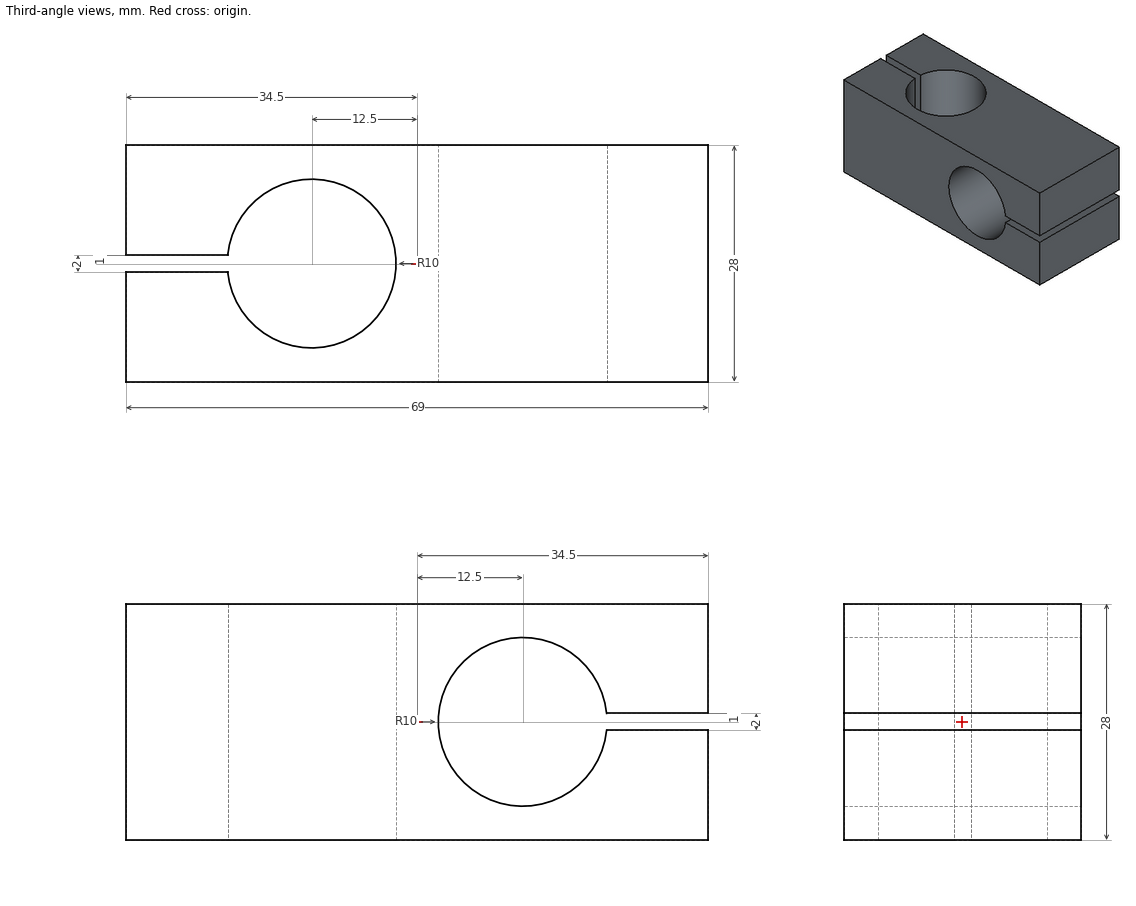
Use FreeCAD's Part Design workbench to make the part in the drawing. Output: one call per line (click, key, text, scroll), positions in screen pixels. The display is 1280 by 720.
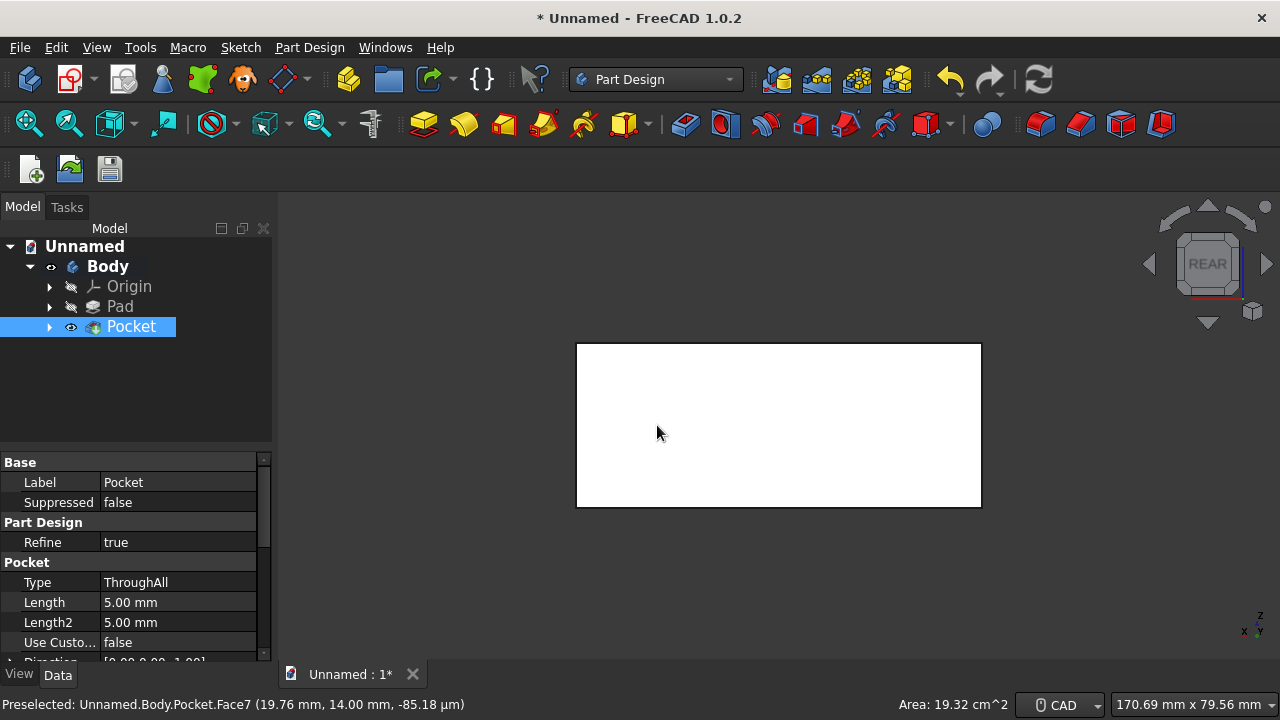
click(70, 80)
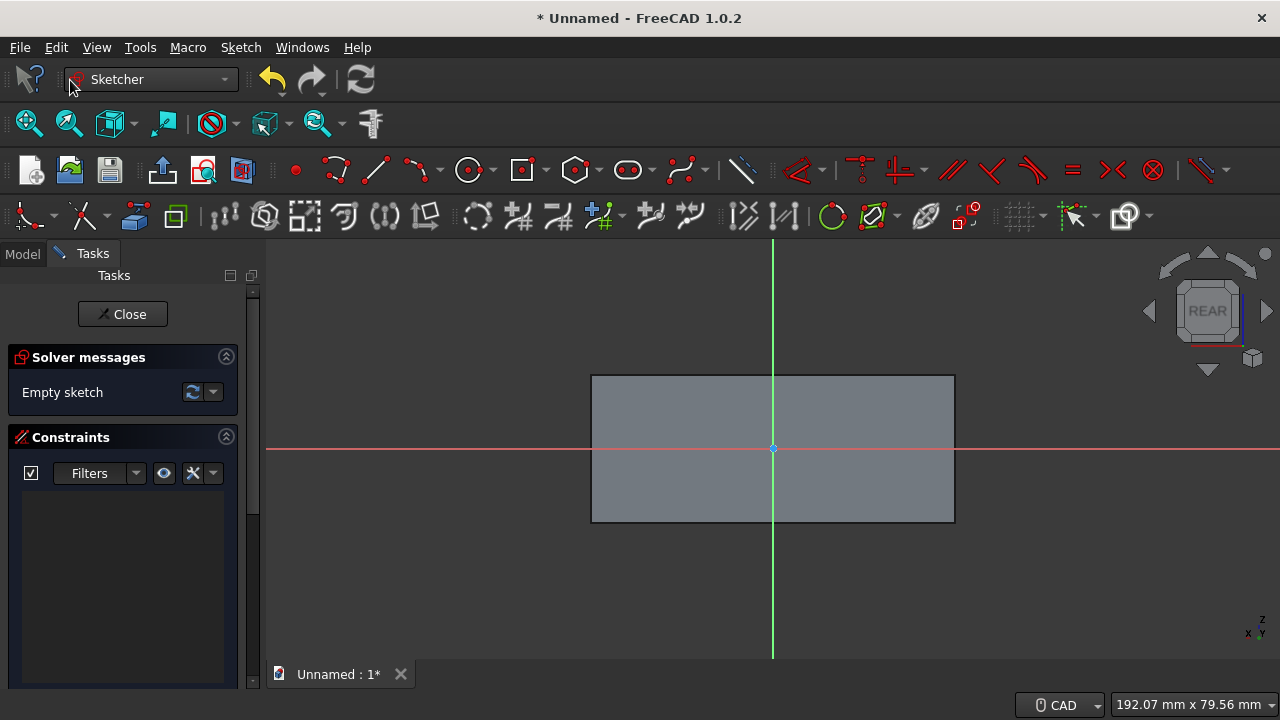
scroll(672, 449, up, 6)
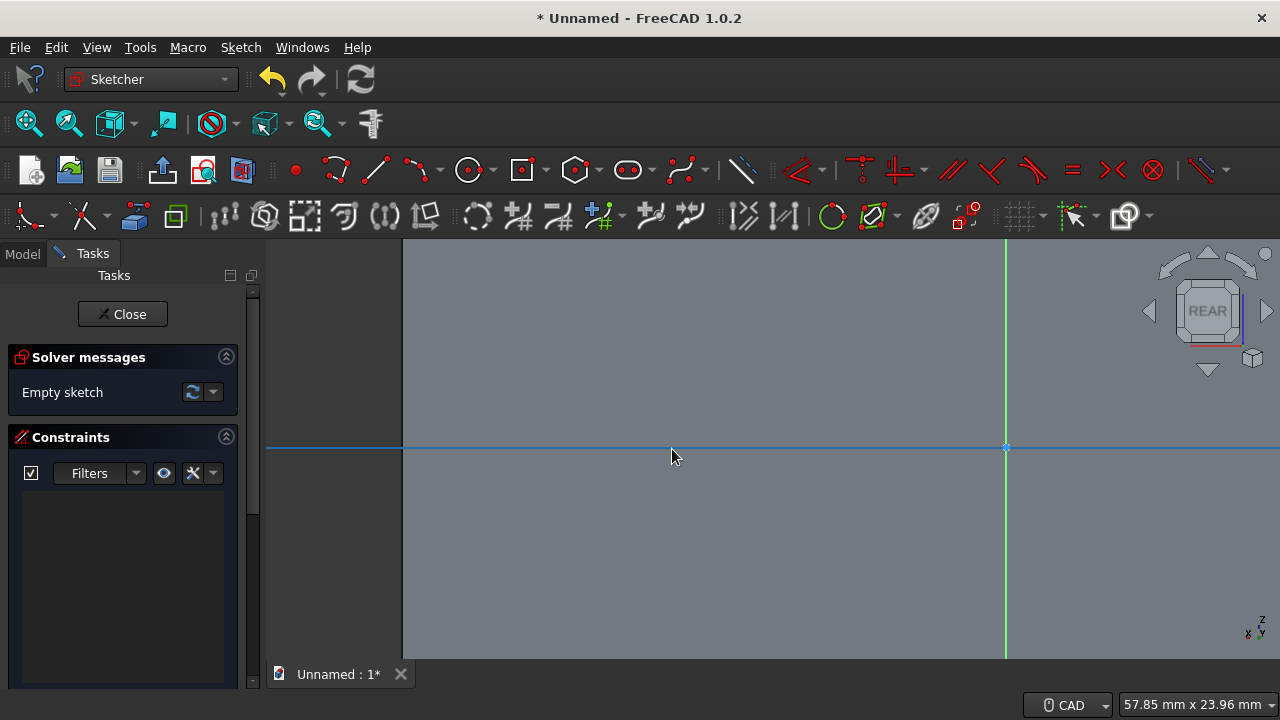
key(g)
key(m)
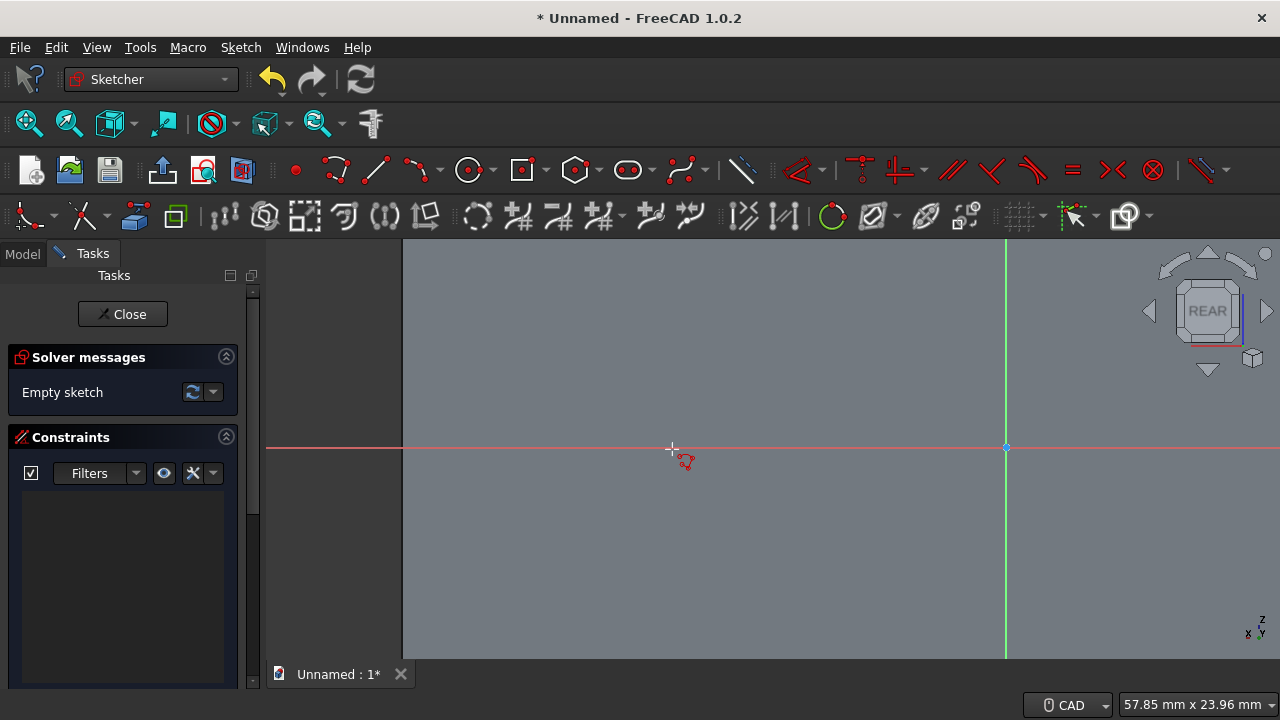
click(613, 430)
click(402, 430)
click(402, 465)
click(613, 465)
right_click(613, 465)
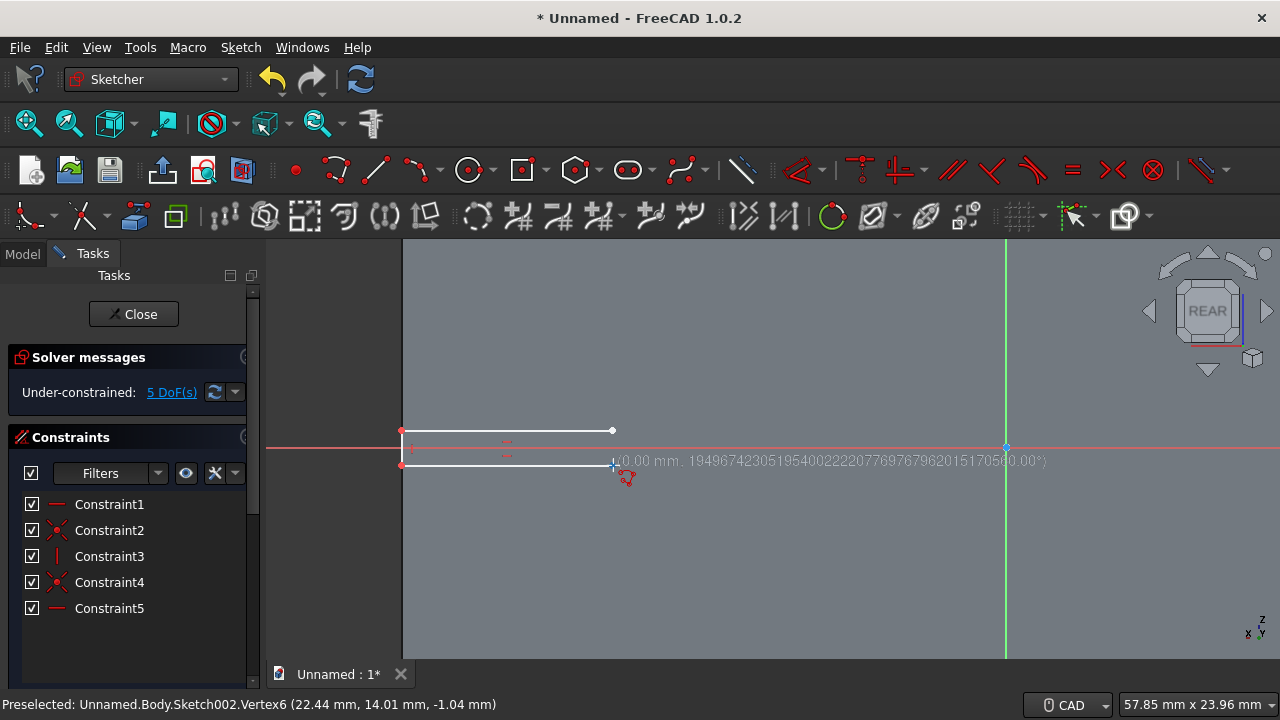
key(g)
key(3)
key(a)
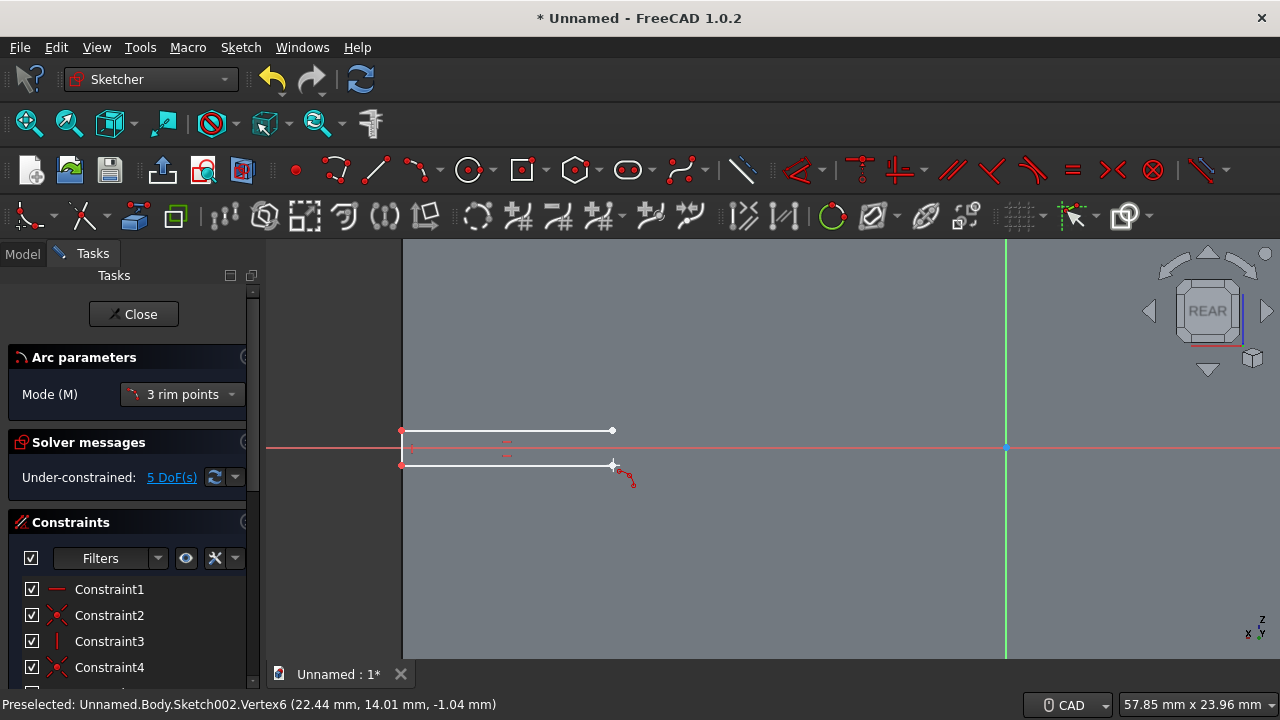
click(613, 466)
click(613, 431)
click(931, 548)
key(Escape)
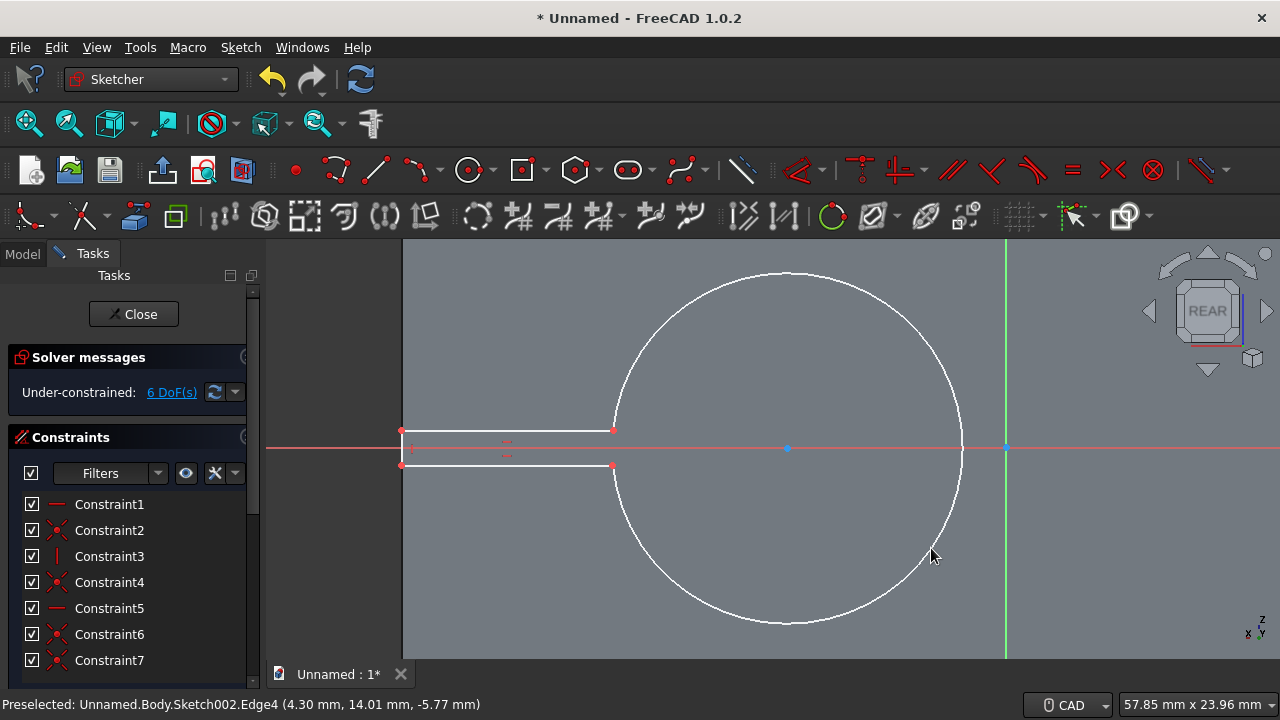
click(787, 449)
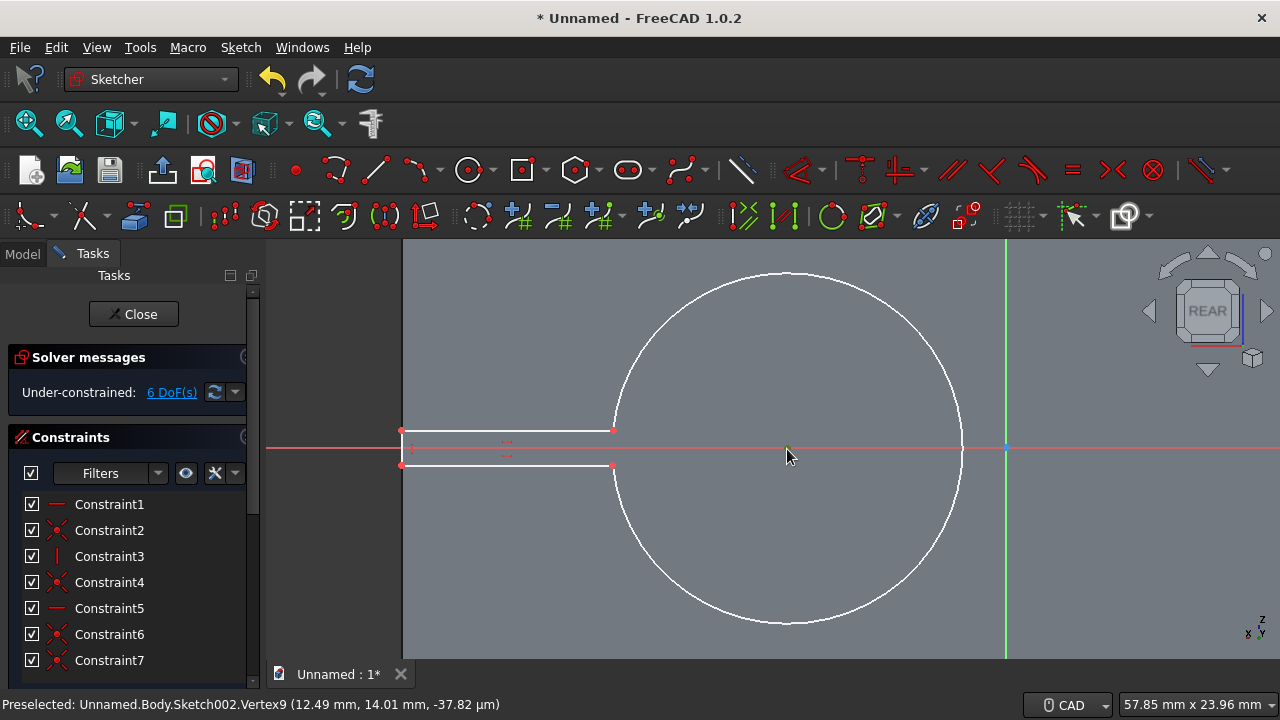
click(353, 448)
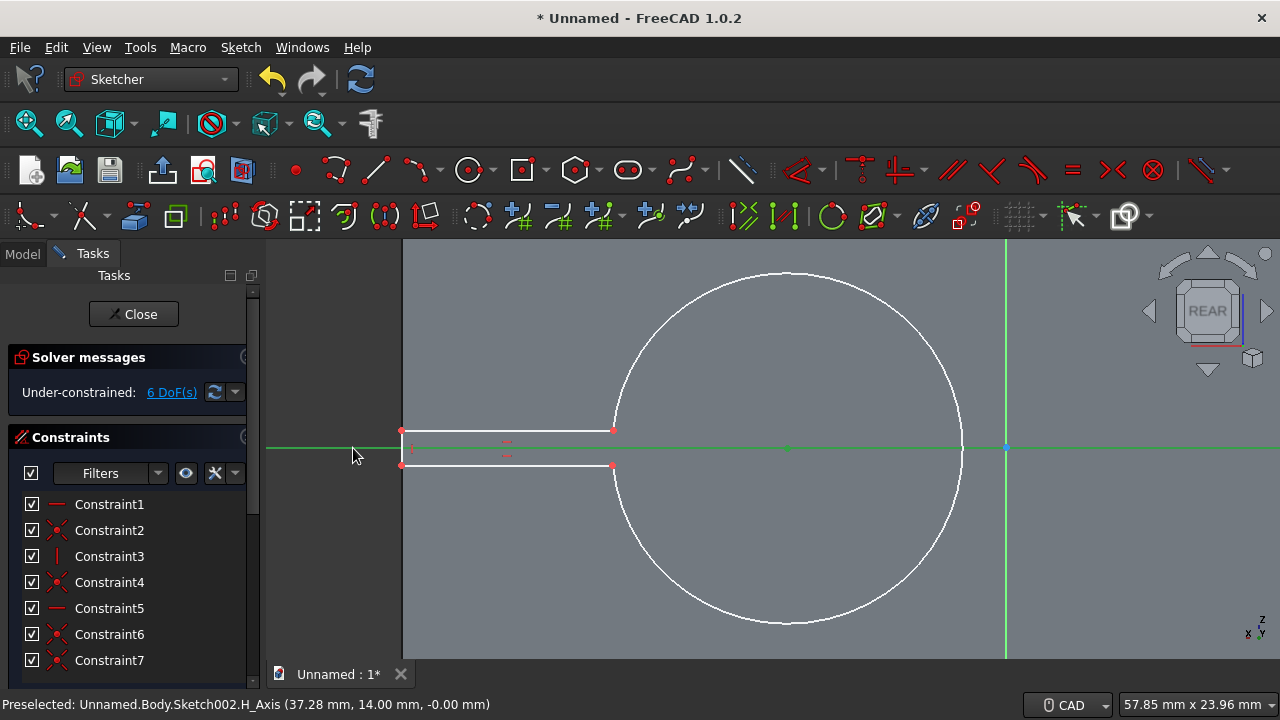
click(860, 170)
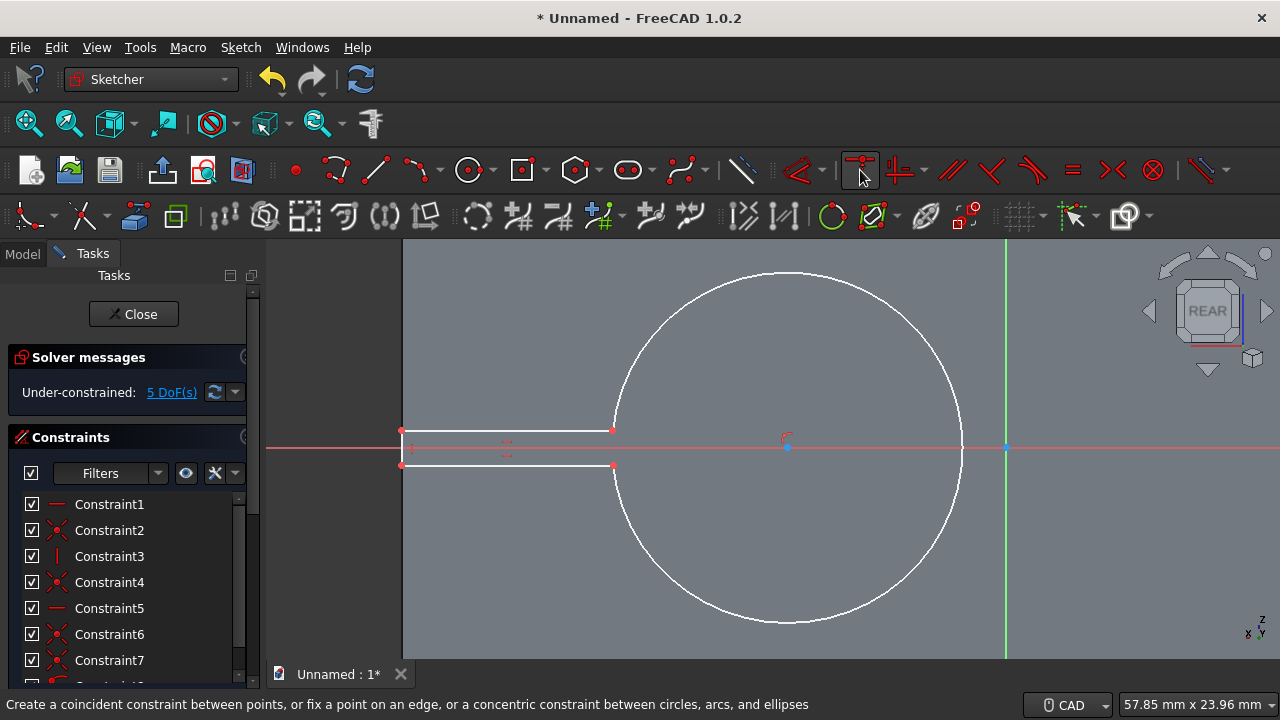
key(d)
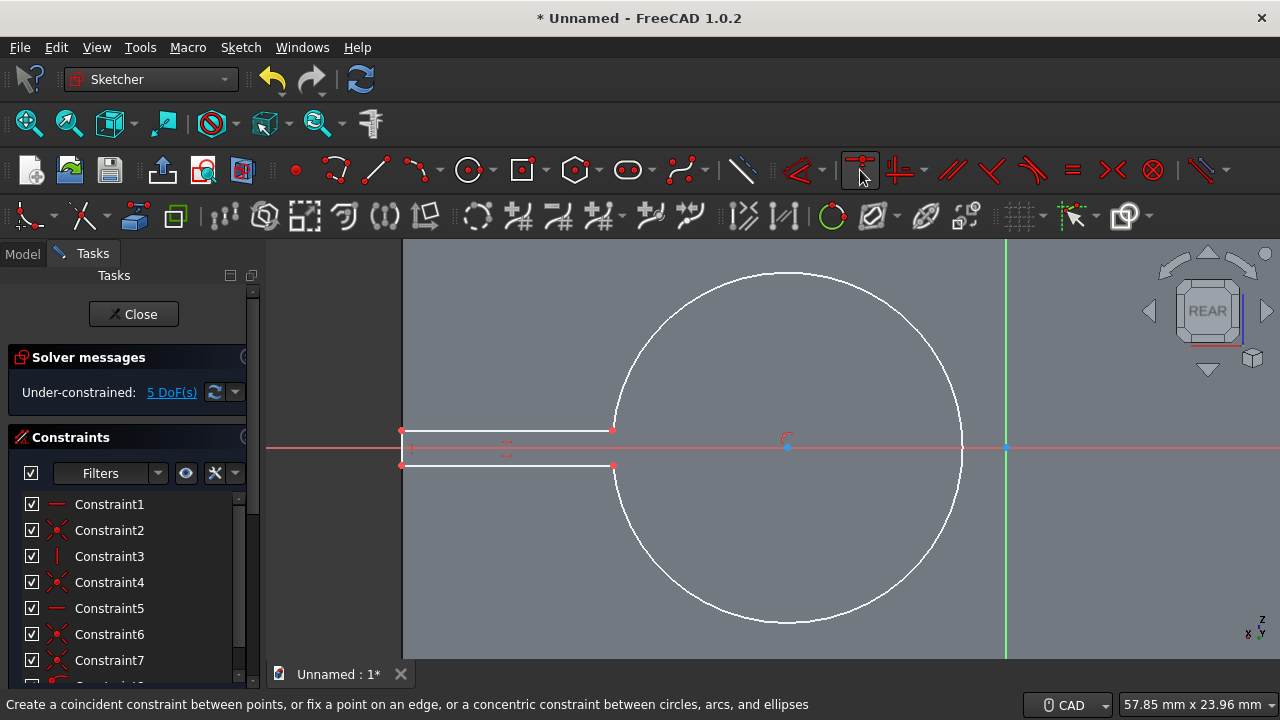
click(849, 612)
click(944, 583)